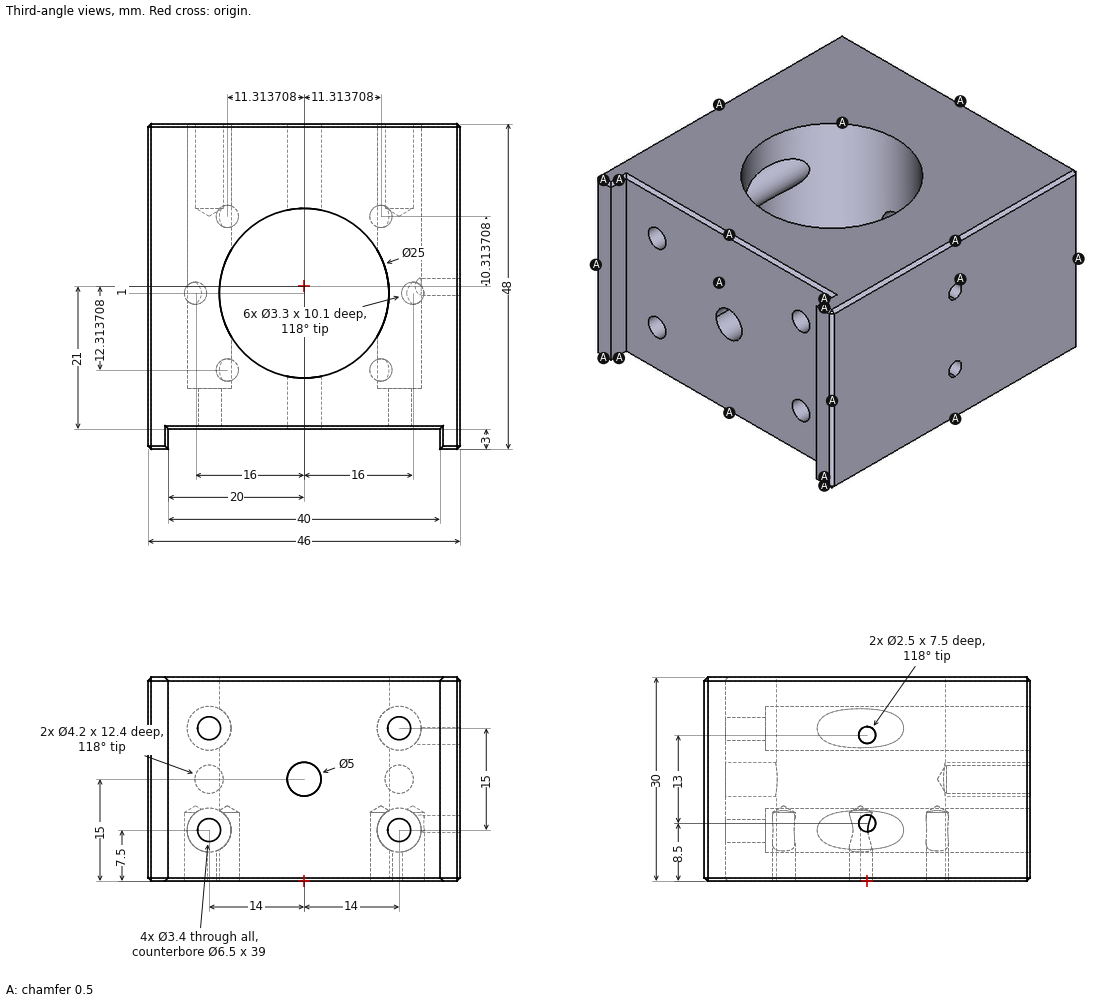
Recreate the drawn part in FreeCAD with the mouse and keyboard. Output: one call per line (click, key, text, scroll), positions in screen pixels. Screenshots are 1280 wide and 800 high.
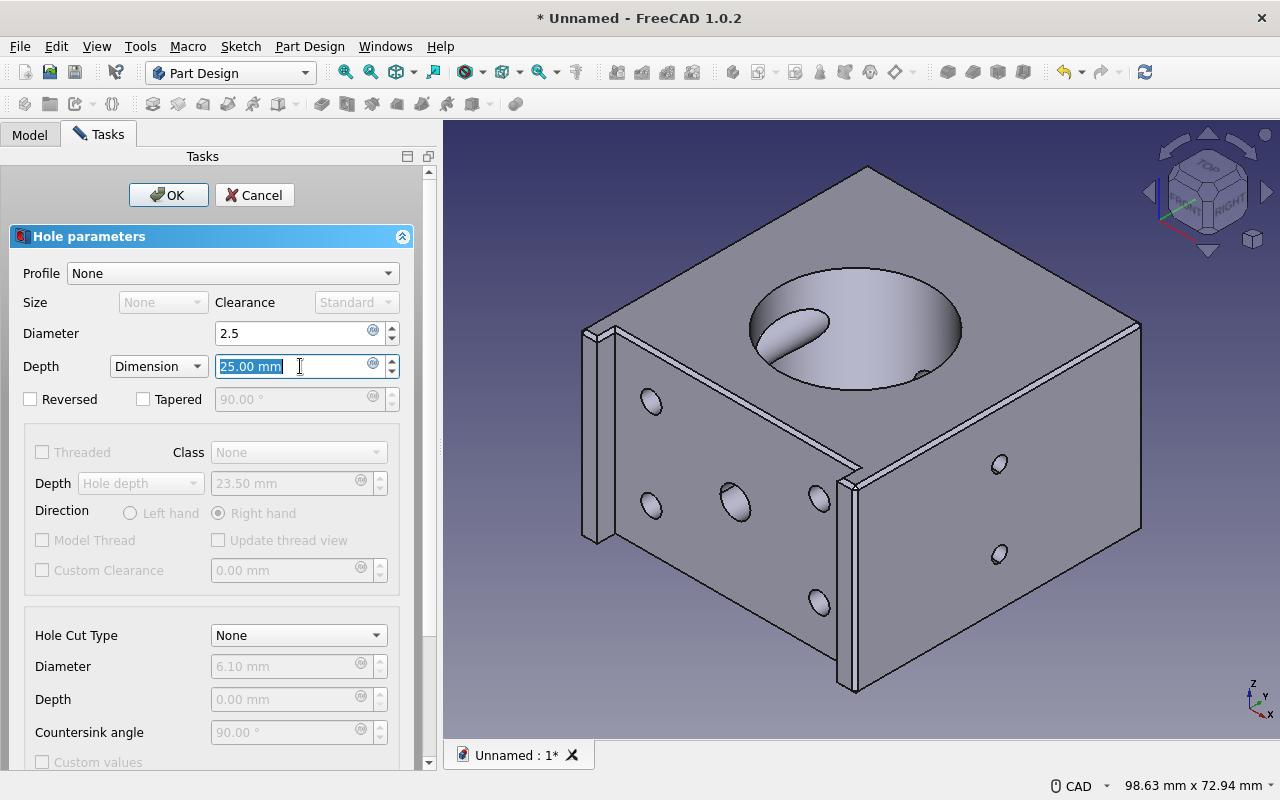
text(7.5)
key(Tab)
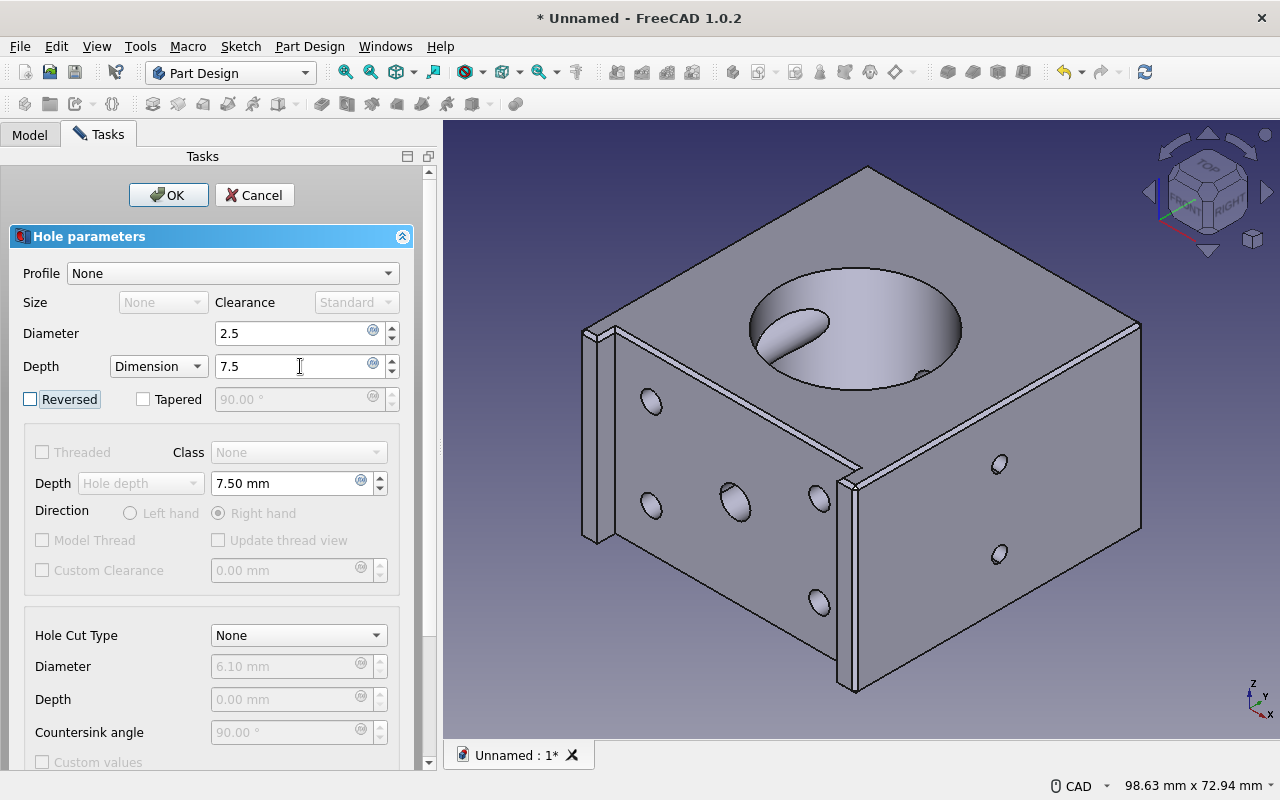
click(169, 195)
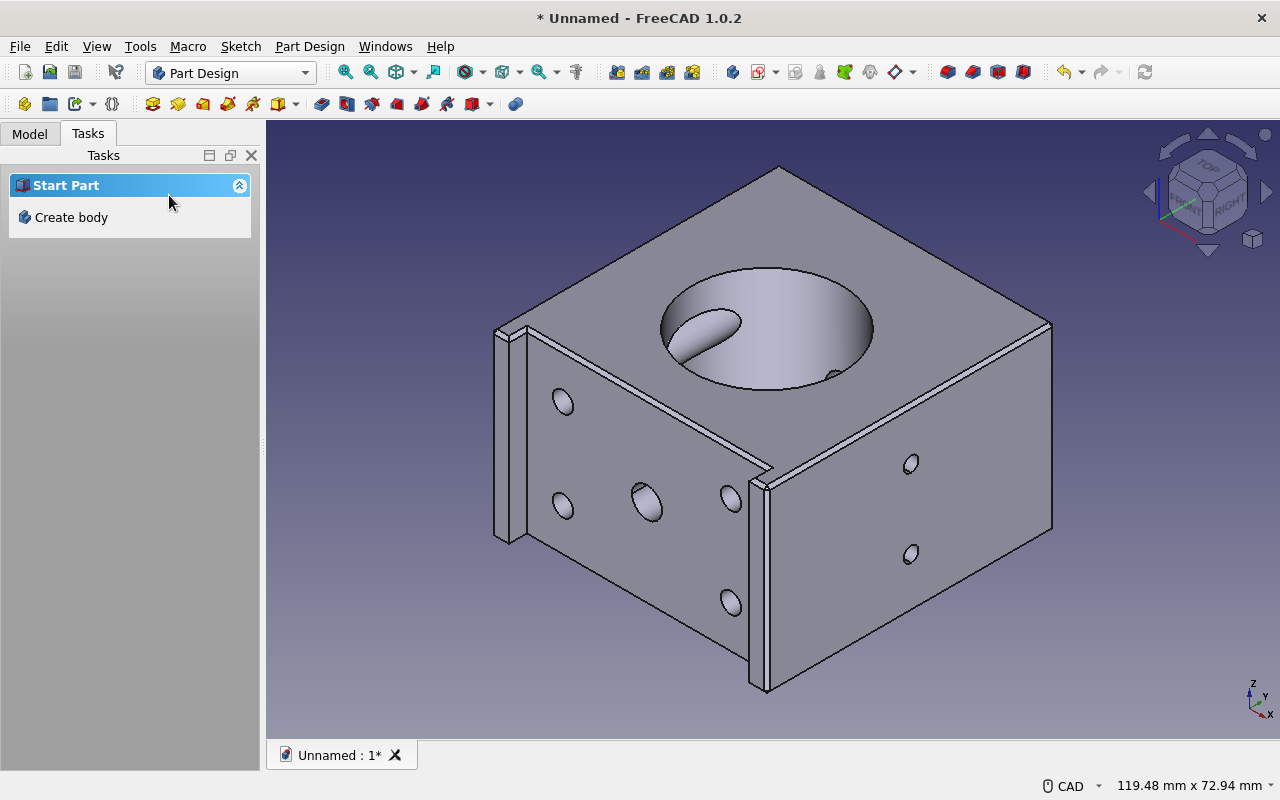
key(5)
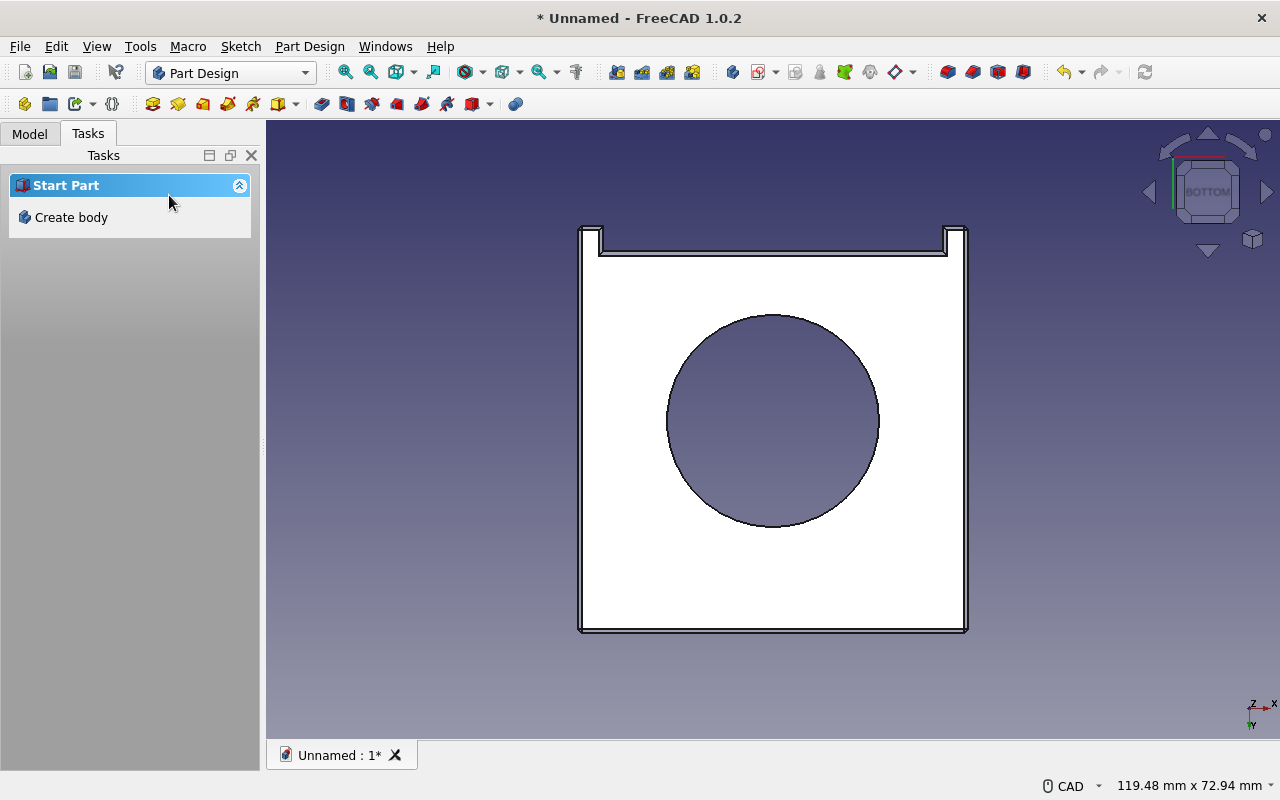
click(664, 542)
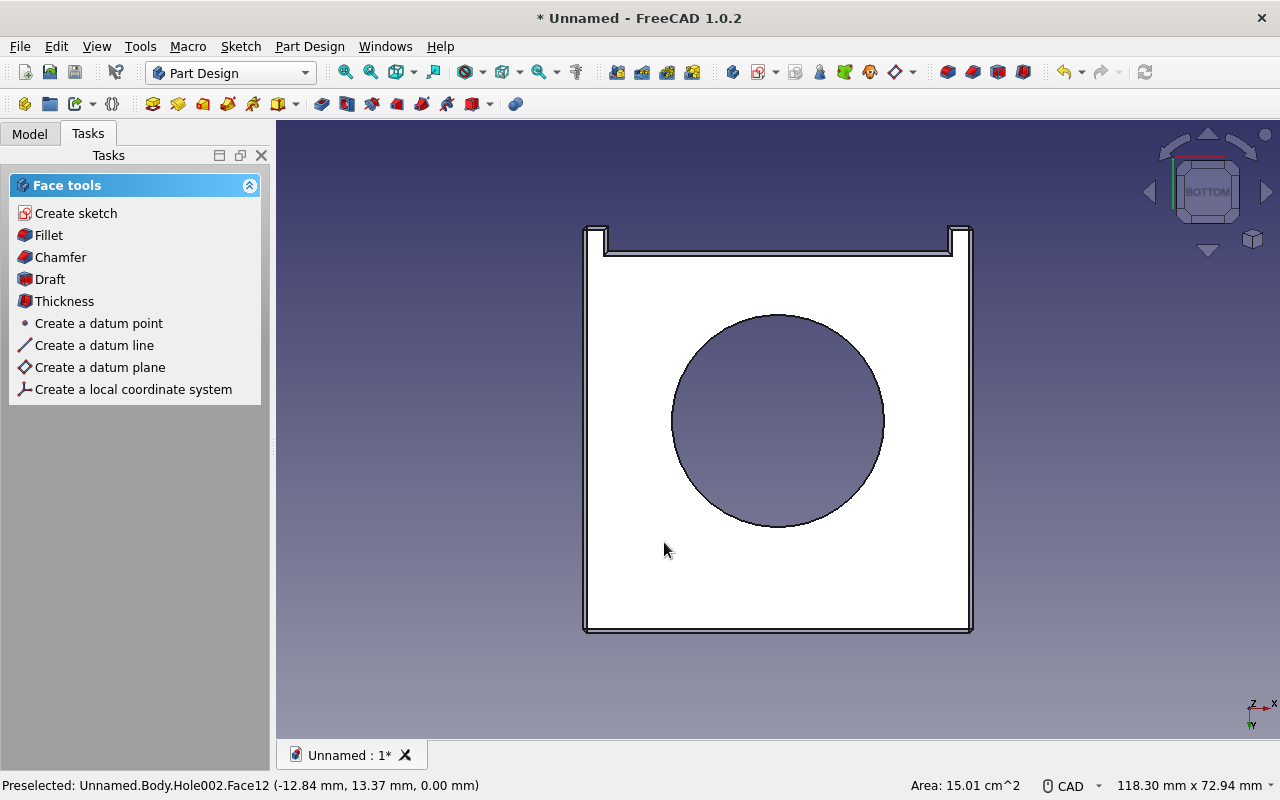
click(758, 72)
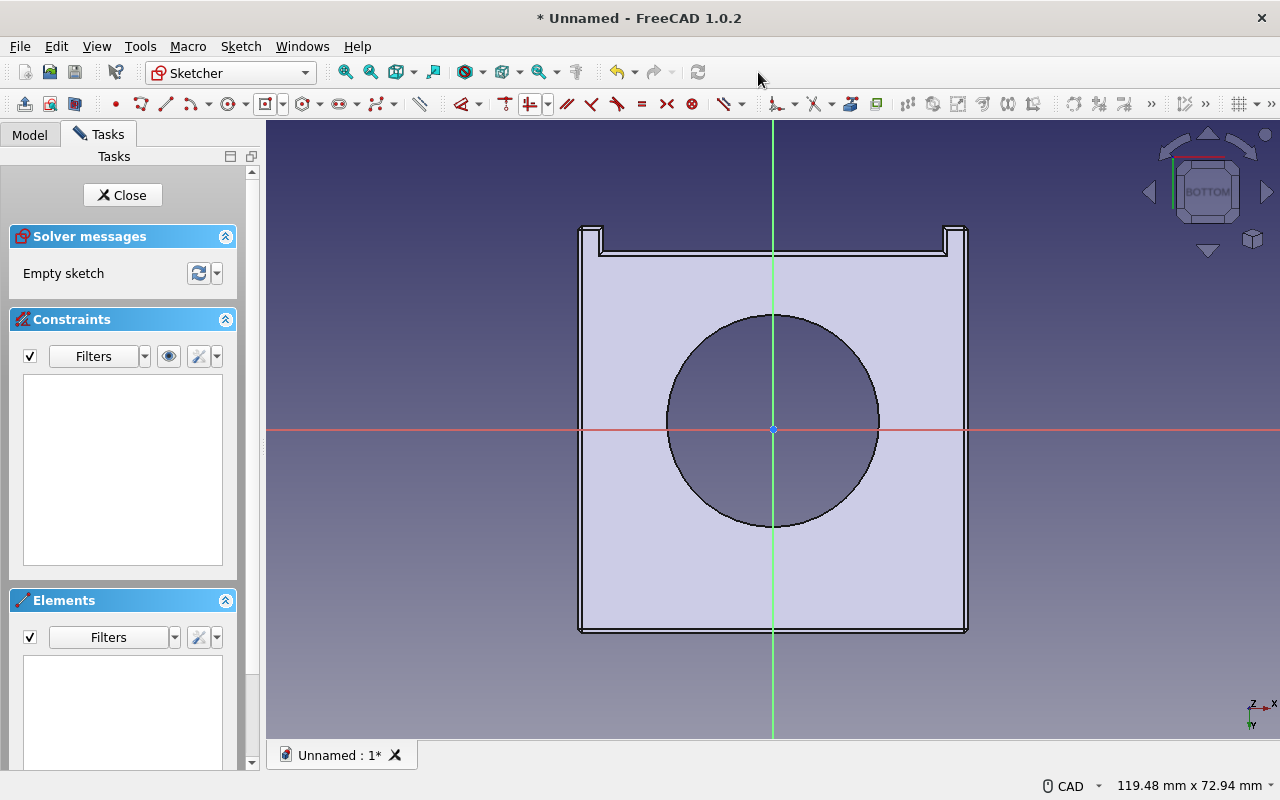
scroll(856, 411, up, 3)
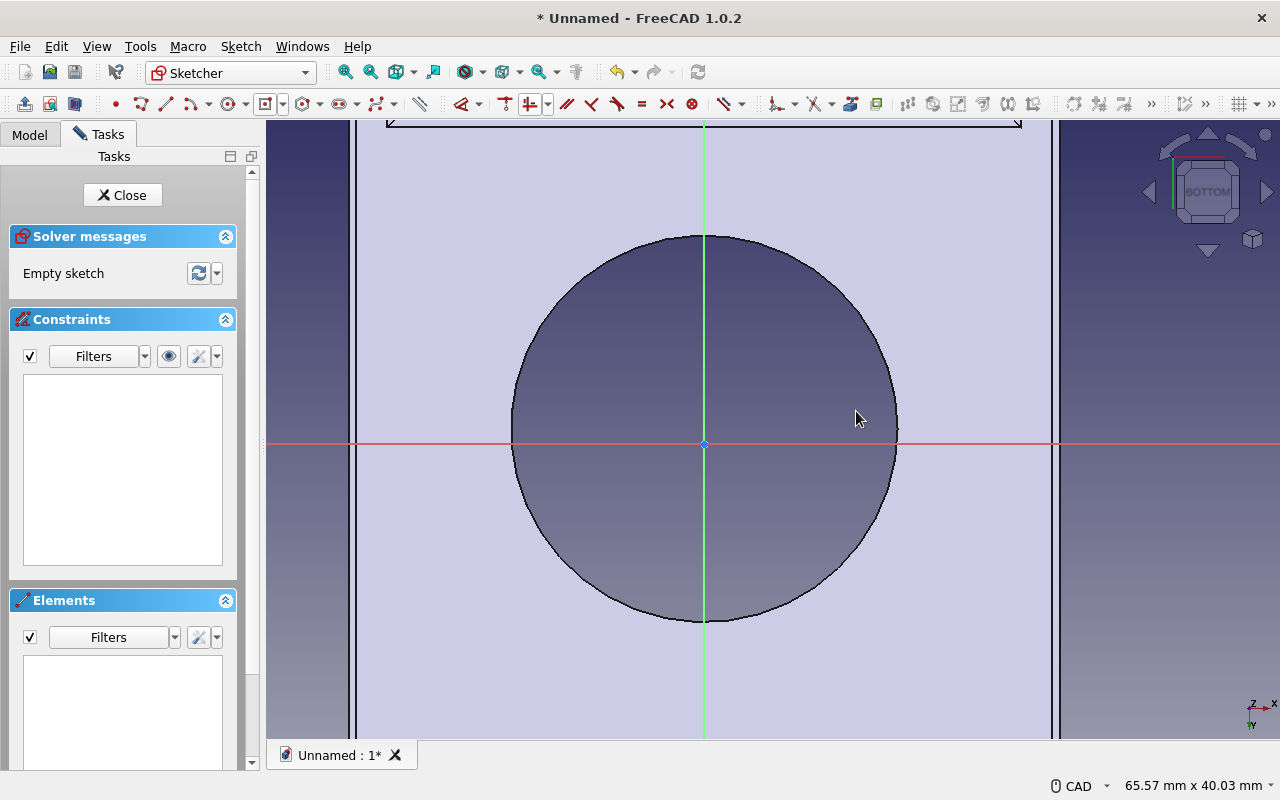
click(228, 104)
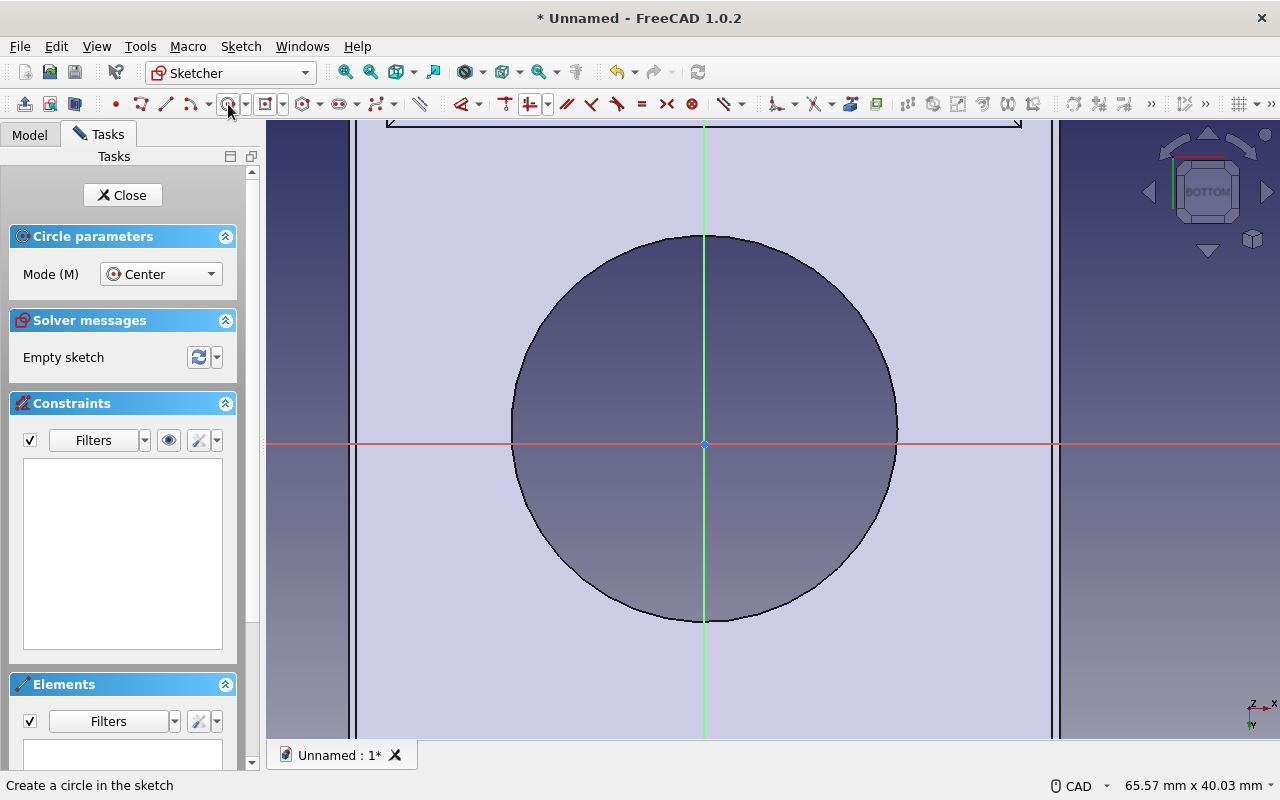
click(952, 429)
move(970, 411)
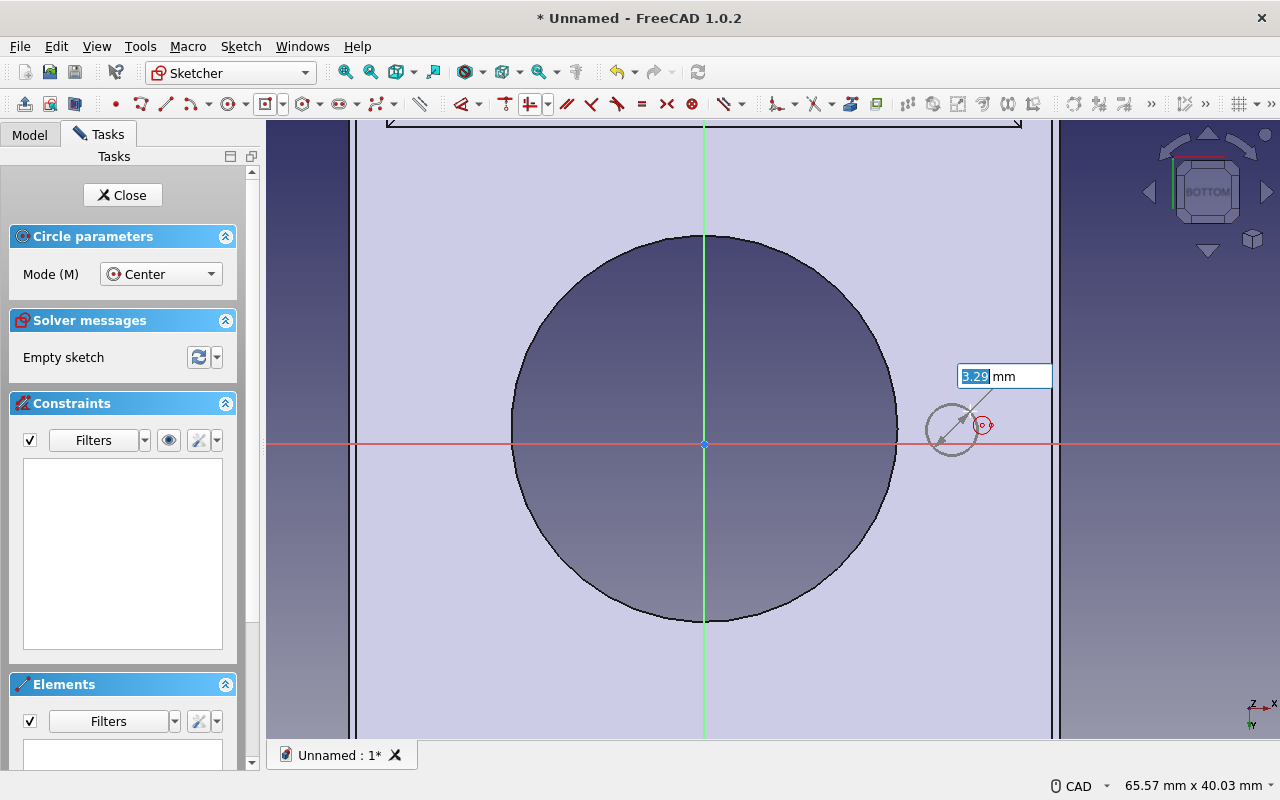
text(3.3)
key(Return)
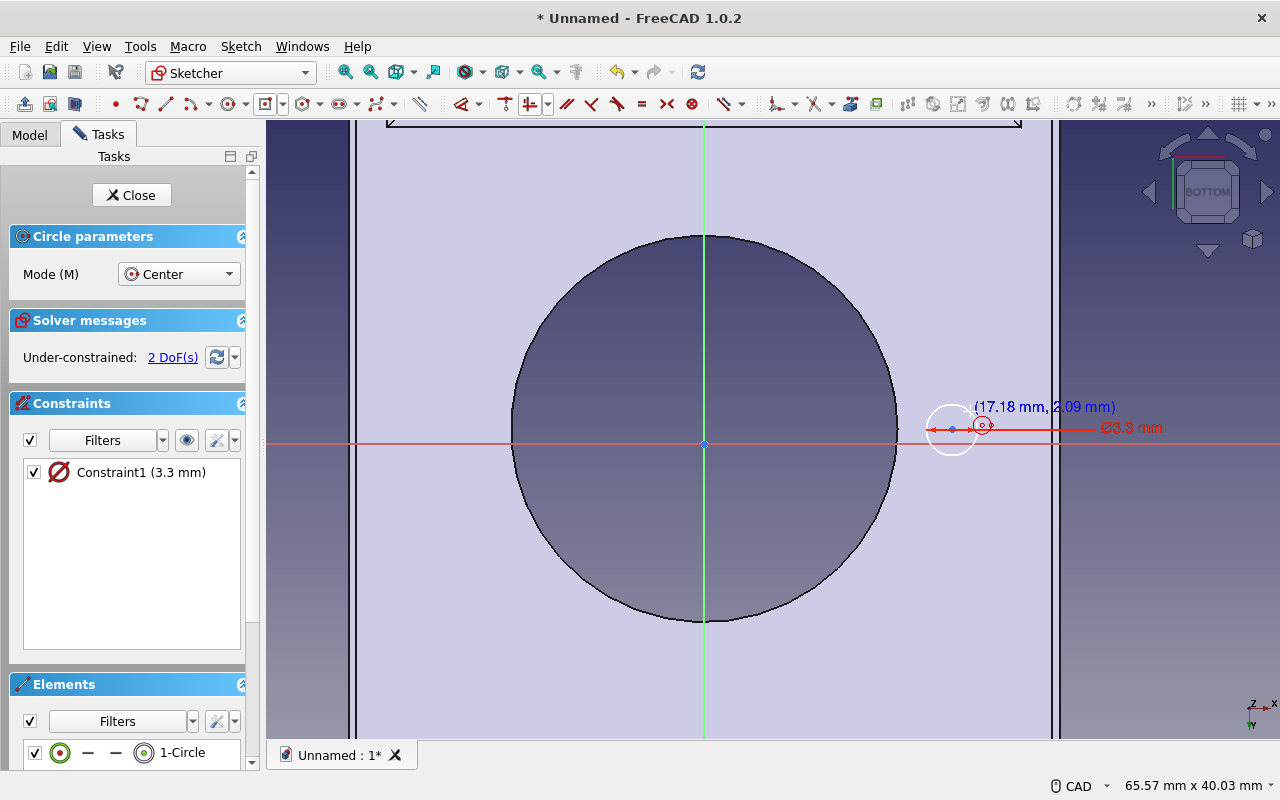
click(879, 604)
move(897, 586)